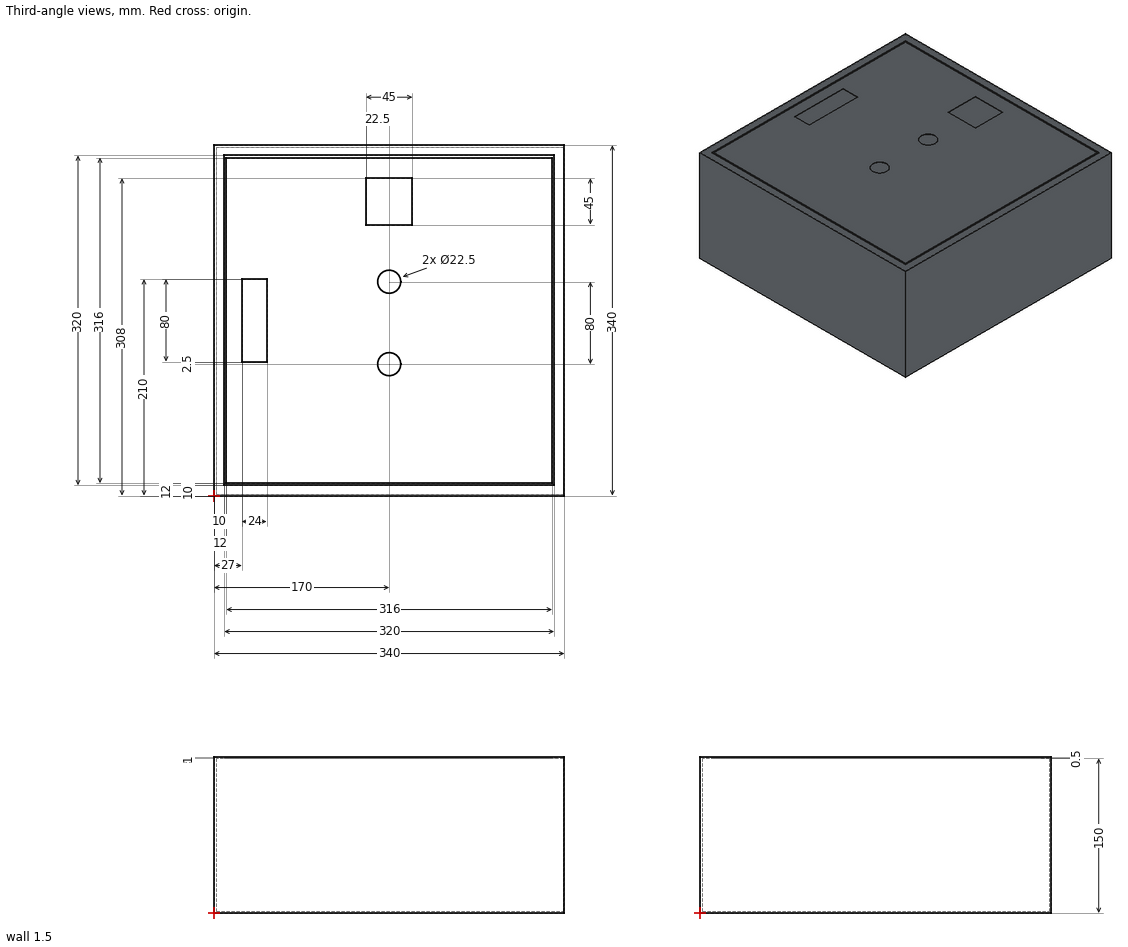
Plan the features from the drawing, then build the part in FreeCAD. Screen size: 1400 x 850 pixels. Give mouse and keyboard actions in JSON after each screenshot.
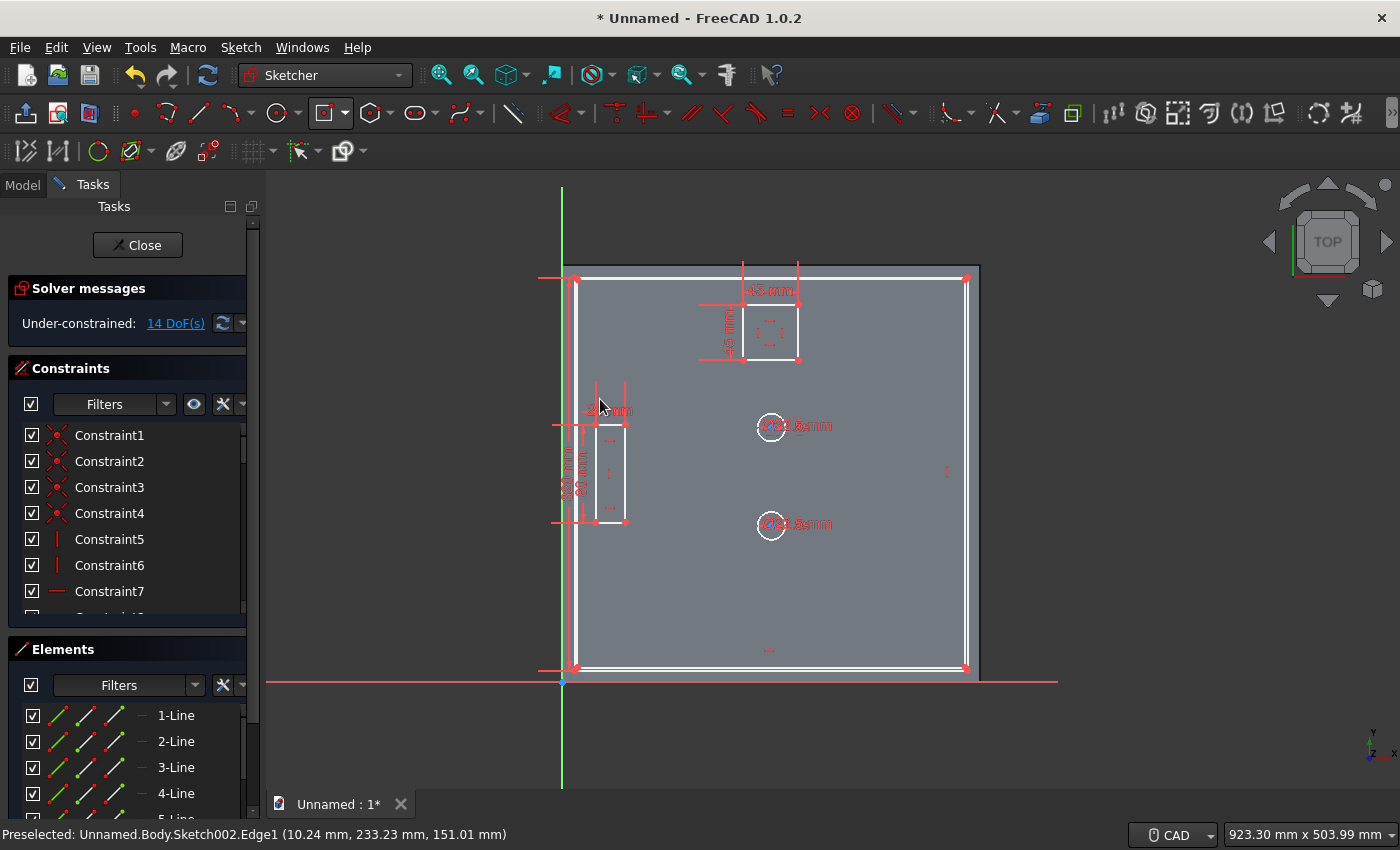
{"action": "scroll", "coordinate": [693, 671], "scroll_direction": "up", "scroll_amount": 8}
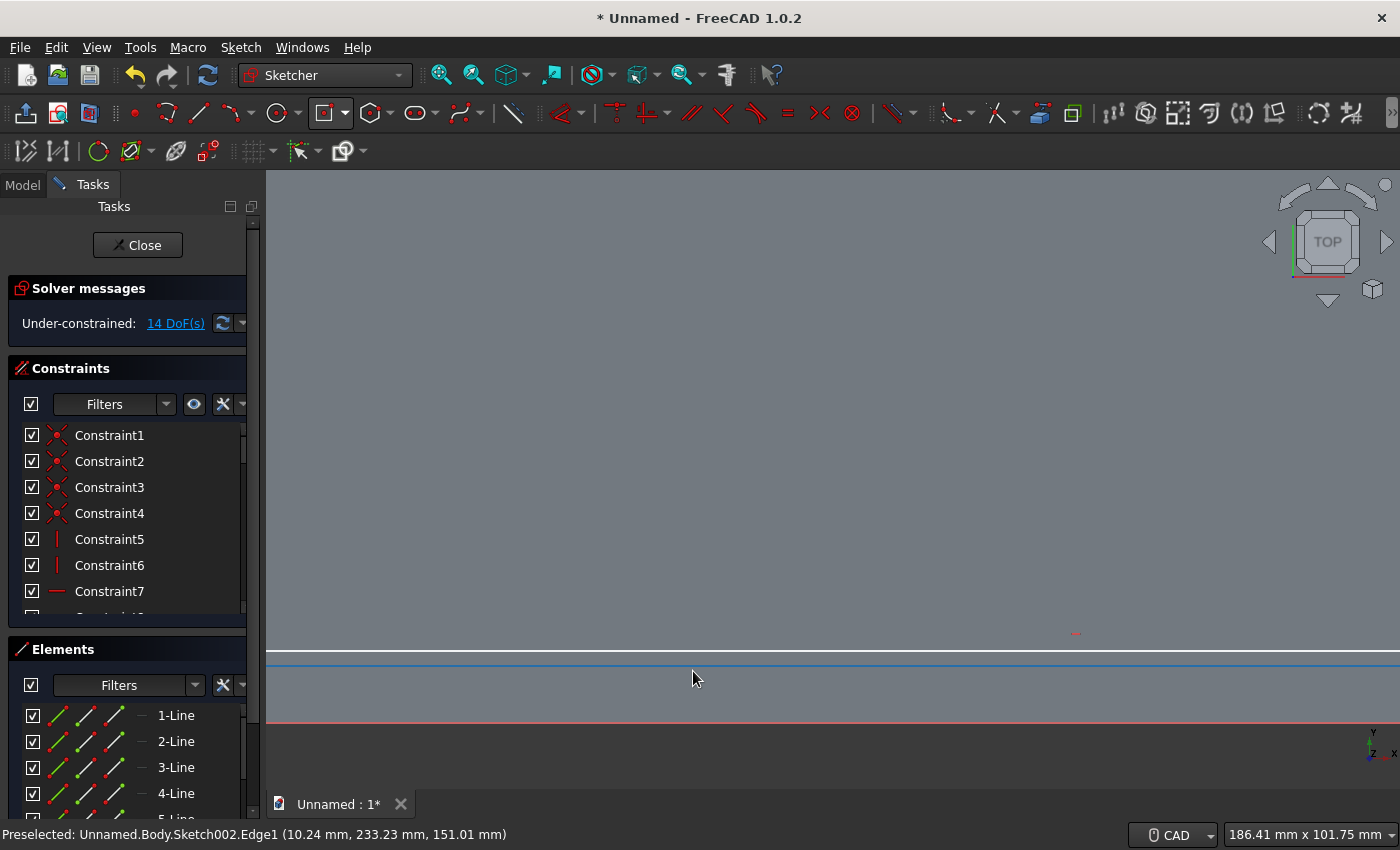
{"action": "left_click", "coordinate": [690, 666]}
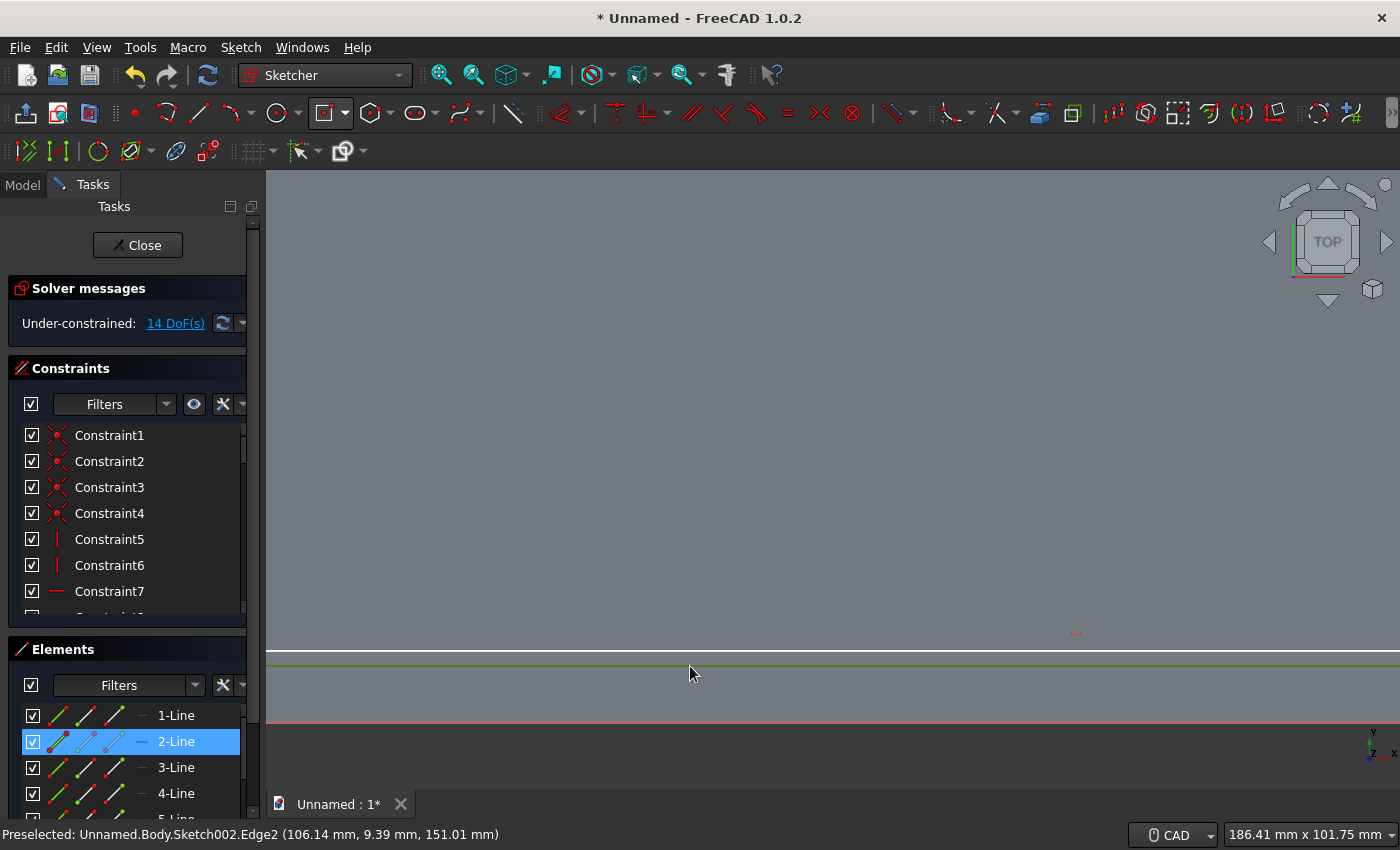
{"action": "key", "text": "l"}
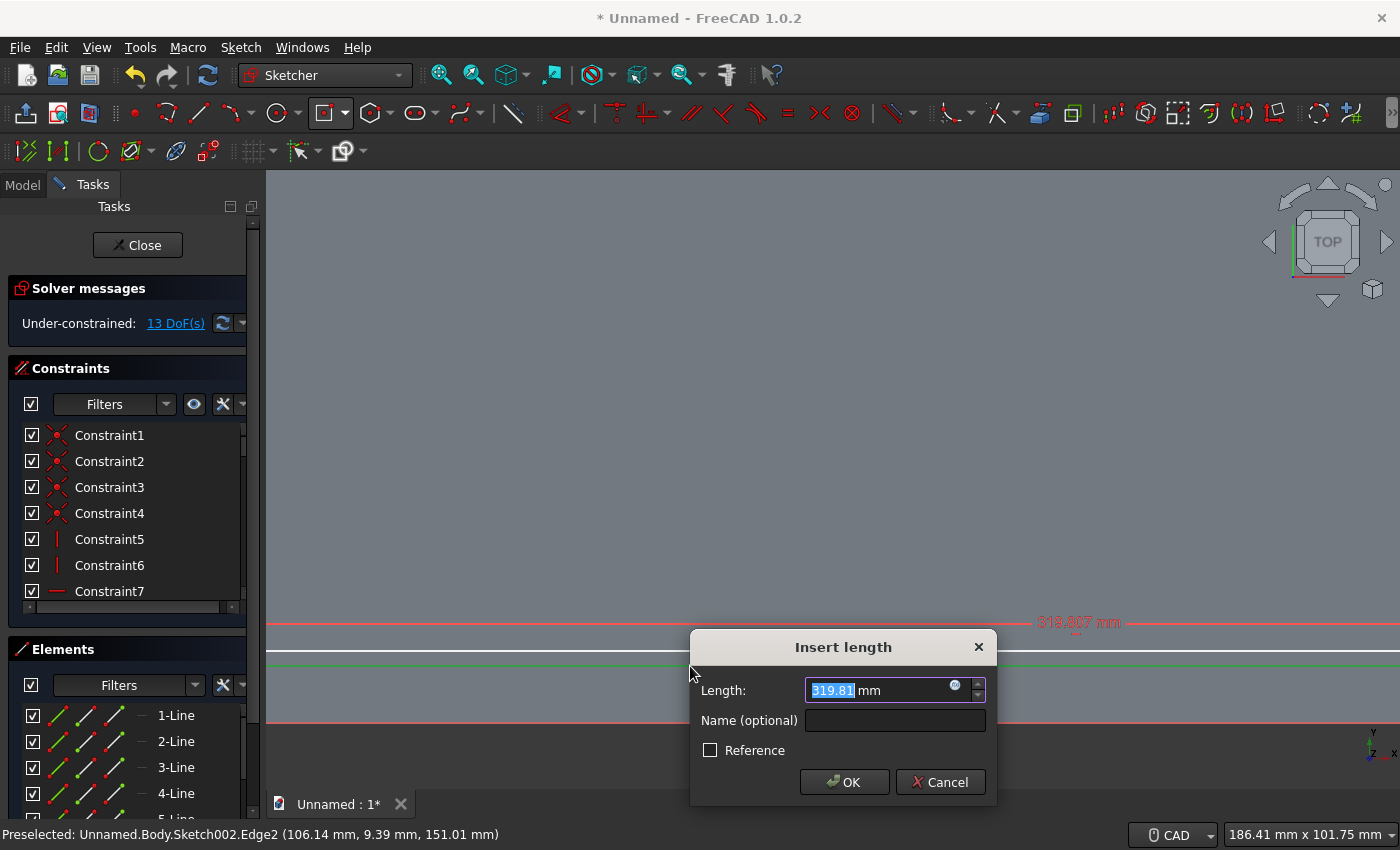
{"action": "type", "text": "320"}
{"action": "key", "text": "Return"}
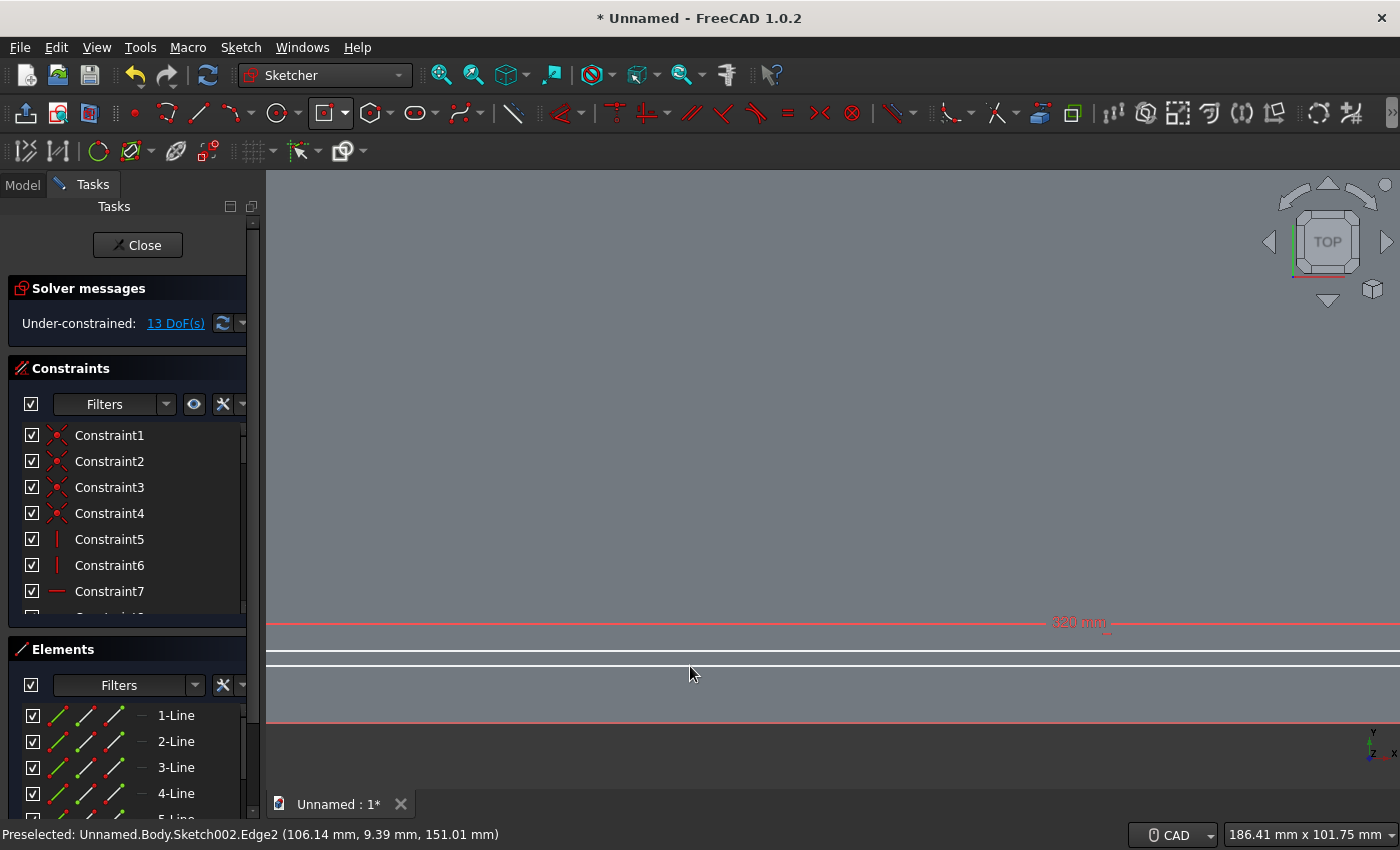
{"action": "scroll", "coordinate": [693, 672], "scroll_direction": "down", "scroll_amount": 8}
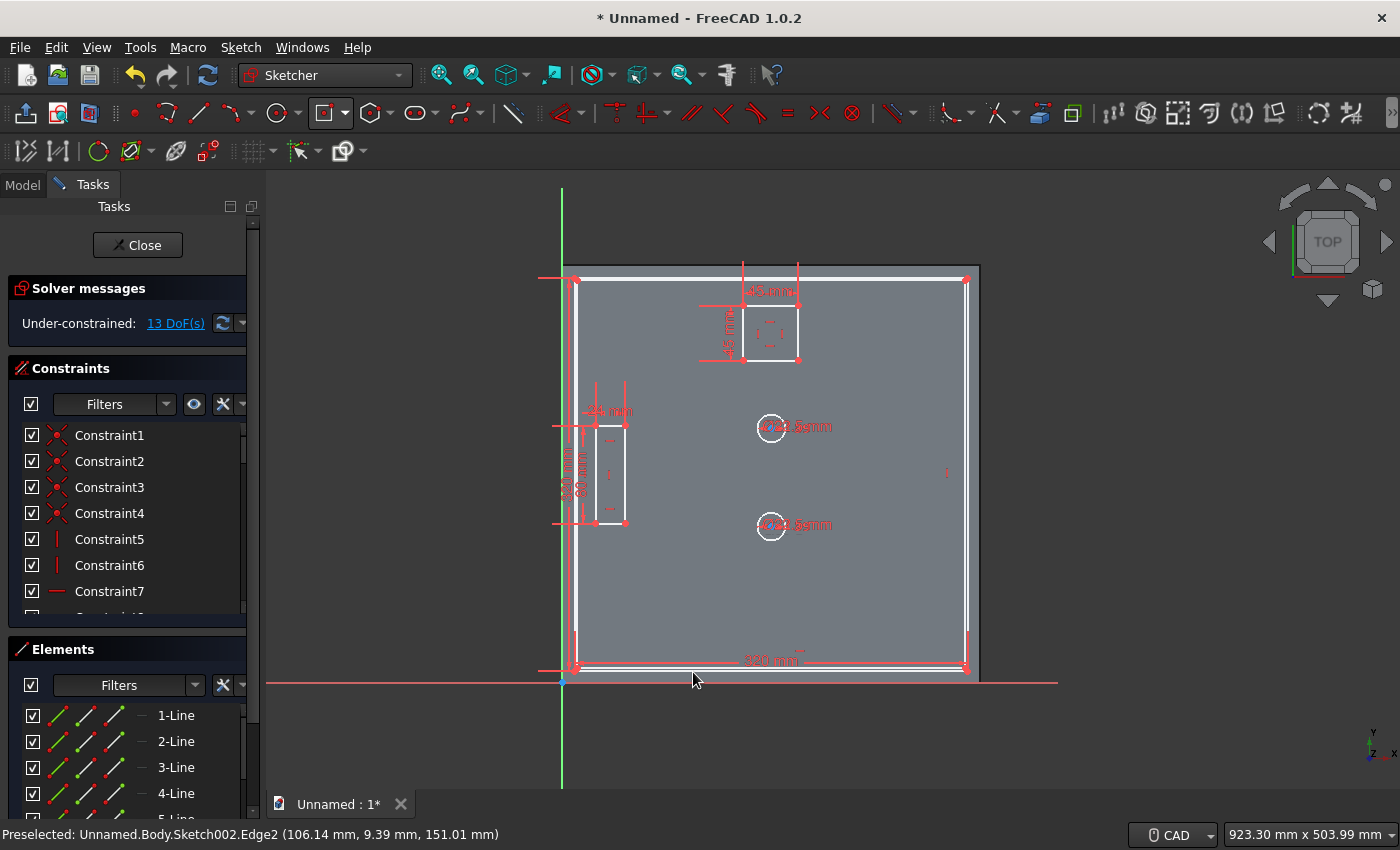
{"action": "scroll", "coordinate": [577, 397], "scroll_direction": "up", "scroll_amount": 9}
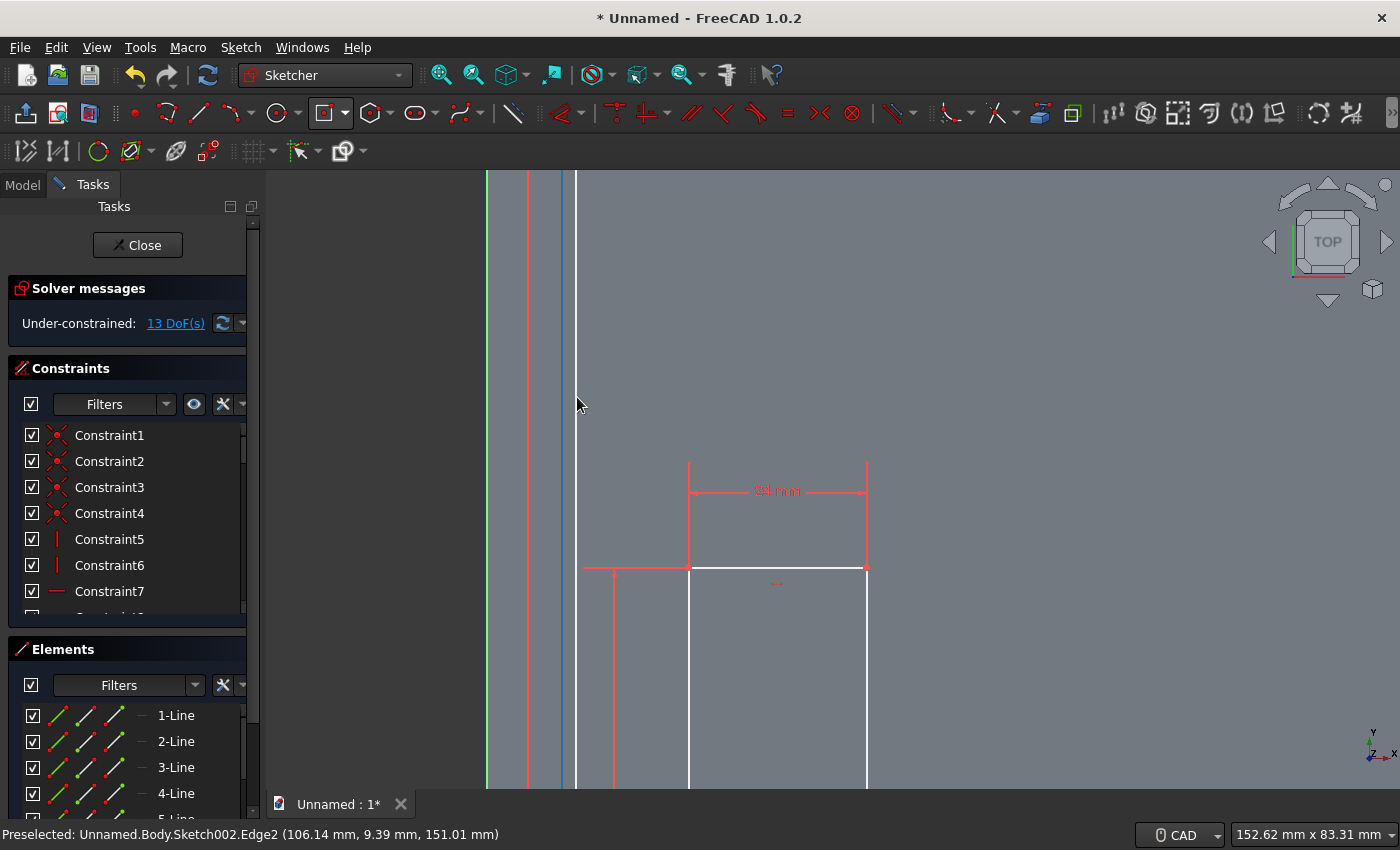
{"action": "left_click", "coordinate": [576, 393]}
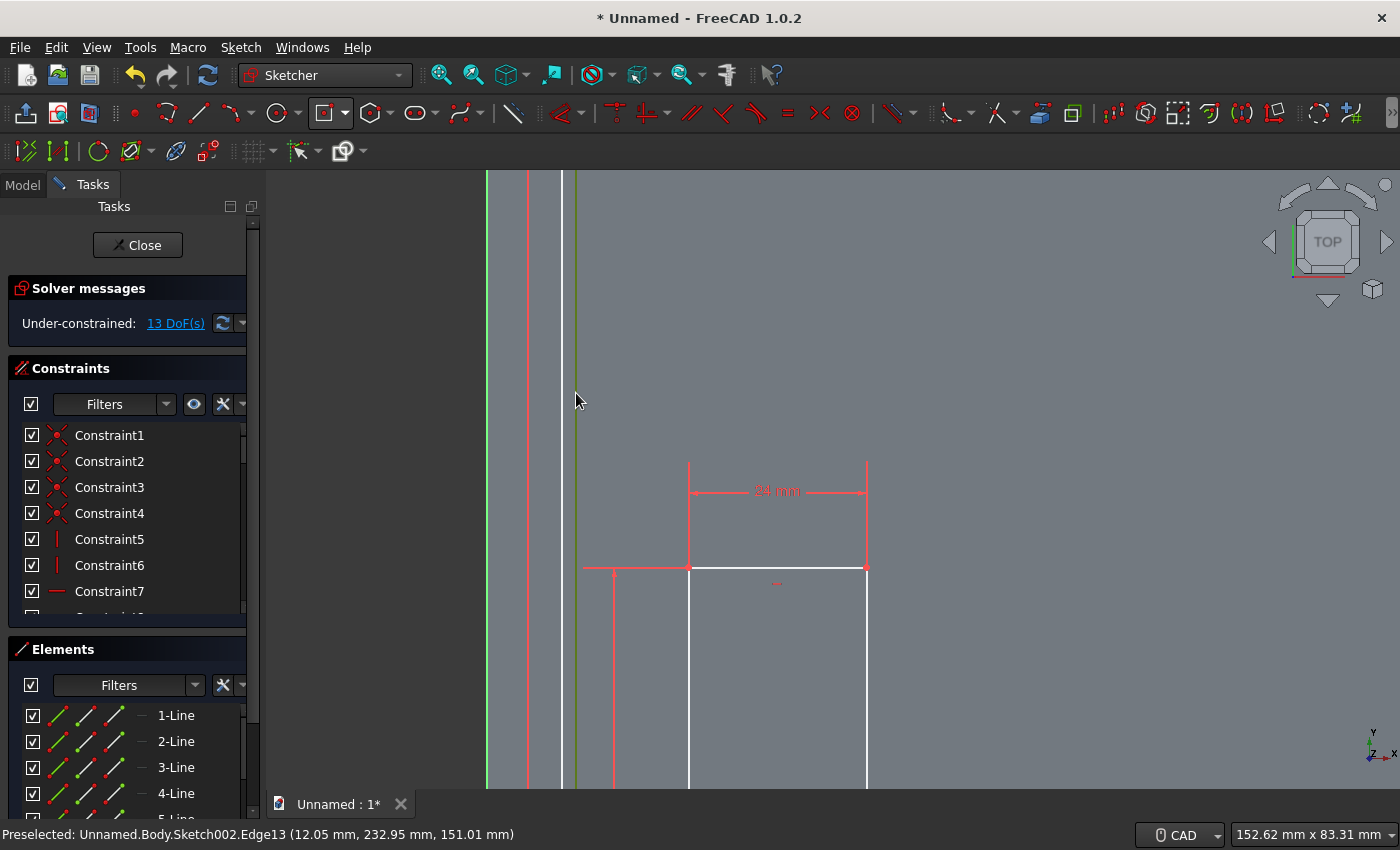
{"action": "key", "text": "i"}